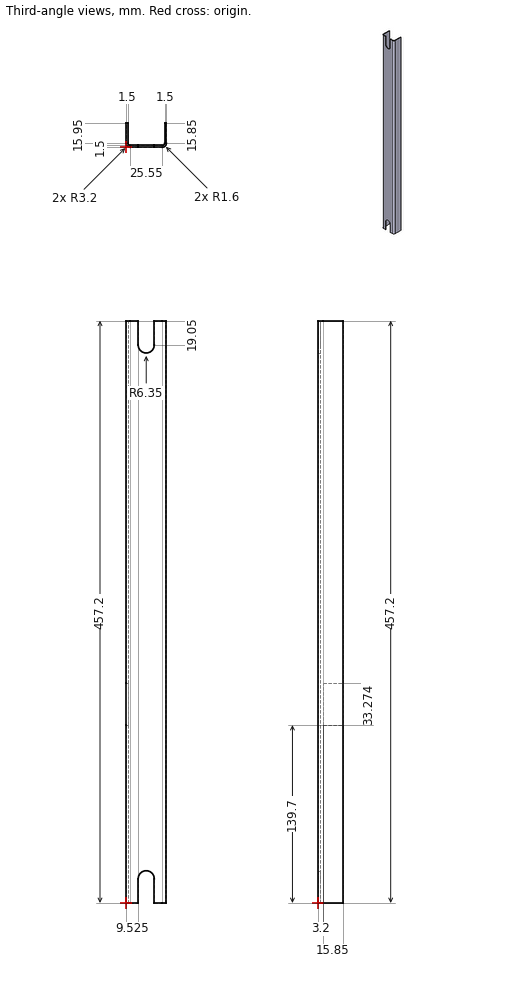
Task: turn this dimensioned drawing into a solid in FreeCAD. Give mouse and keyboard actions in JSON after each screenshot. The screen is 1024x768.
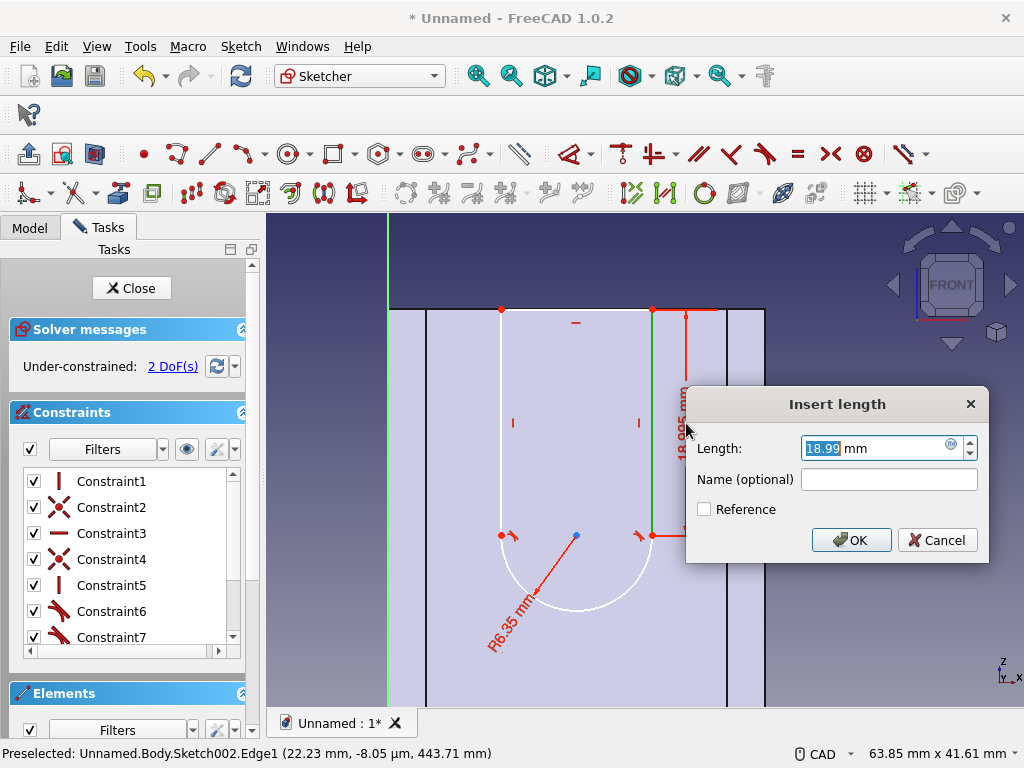
{"action": "type", "text": "19.05"}
{"action": "key", "text": "Return"}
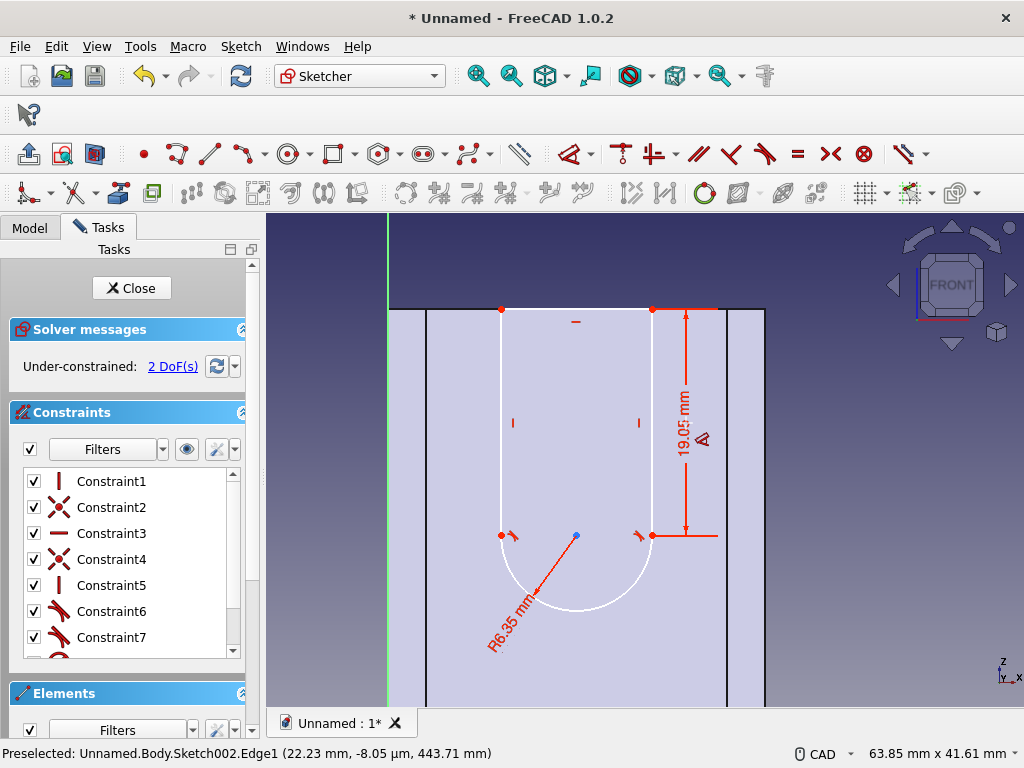
{"action": "left_click", "coordinate": [652, 309]}
{"action": "left_click", "coordinate": [354, 494]}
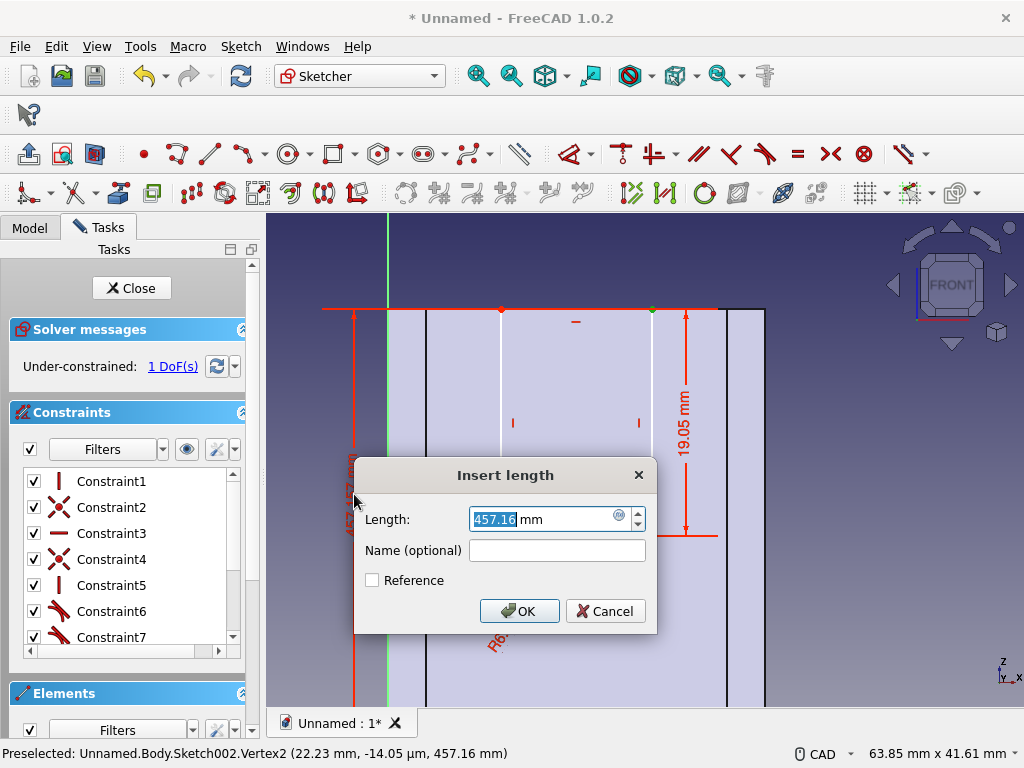
{"action": "type", "text": "457.2"}
{"action": "key", "text": "Return"}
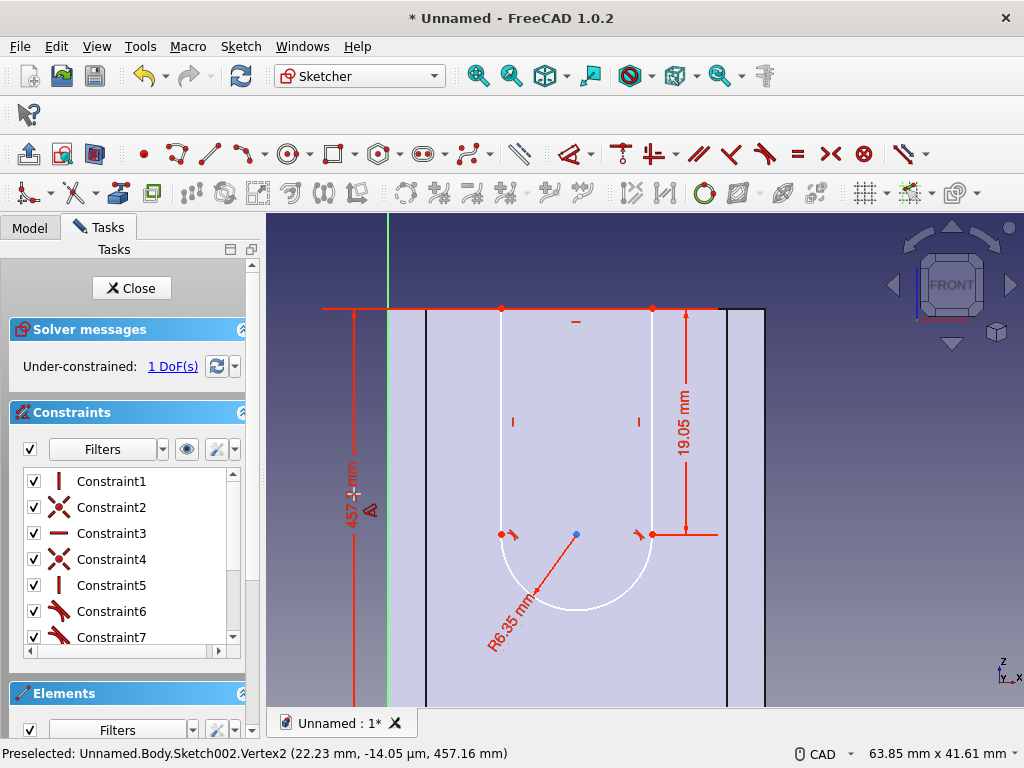
{"action": "left_click", "coordinate": [501, 309]}
{"action": "left_click", "coordinate": [445, 275]}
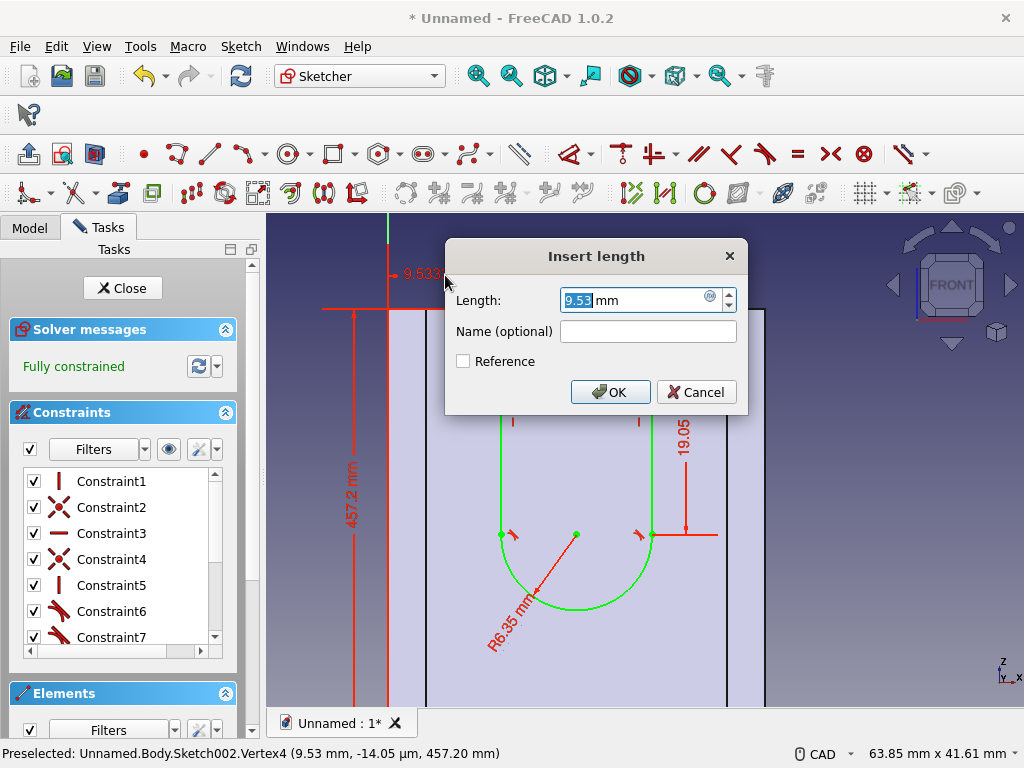
{"action": "type", "text": "9.525"}
{"action": "key", "text": "Return"}
{"action": "key", "text": "Escape"}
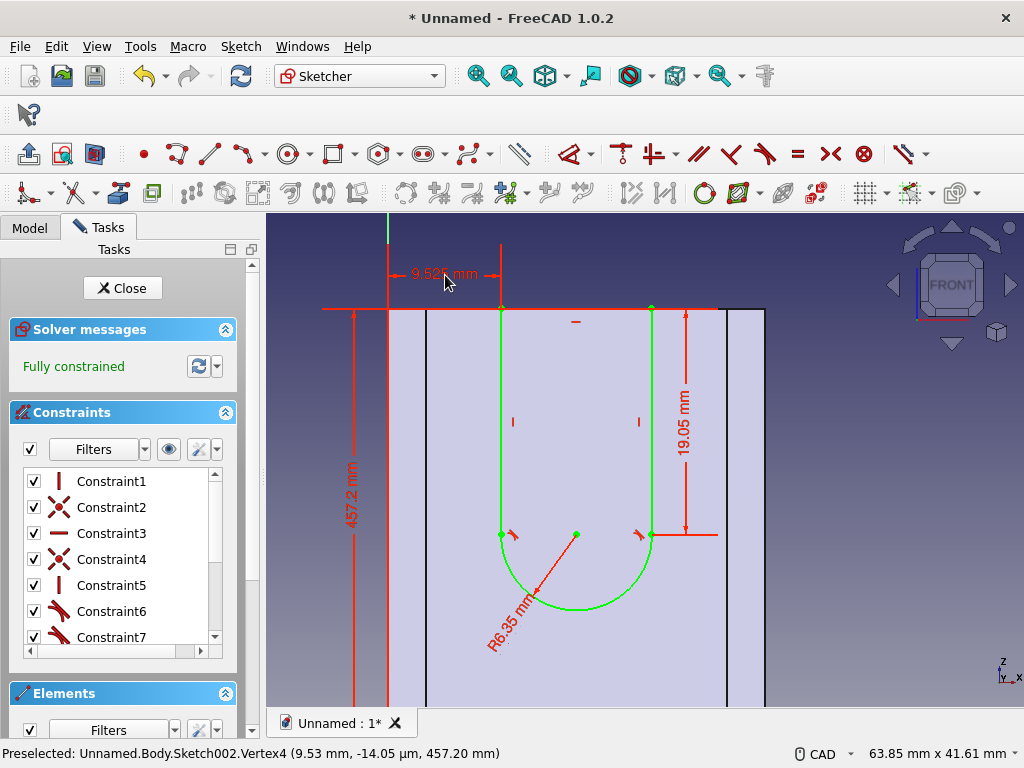
{"action": "left_click", "coordinate": [123, 288]}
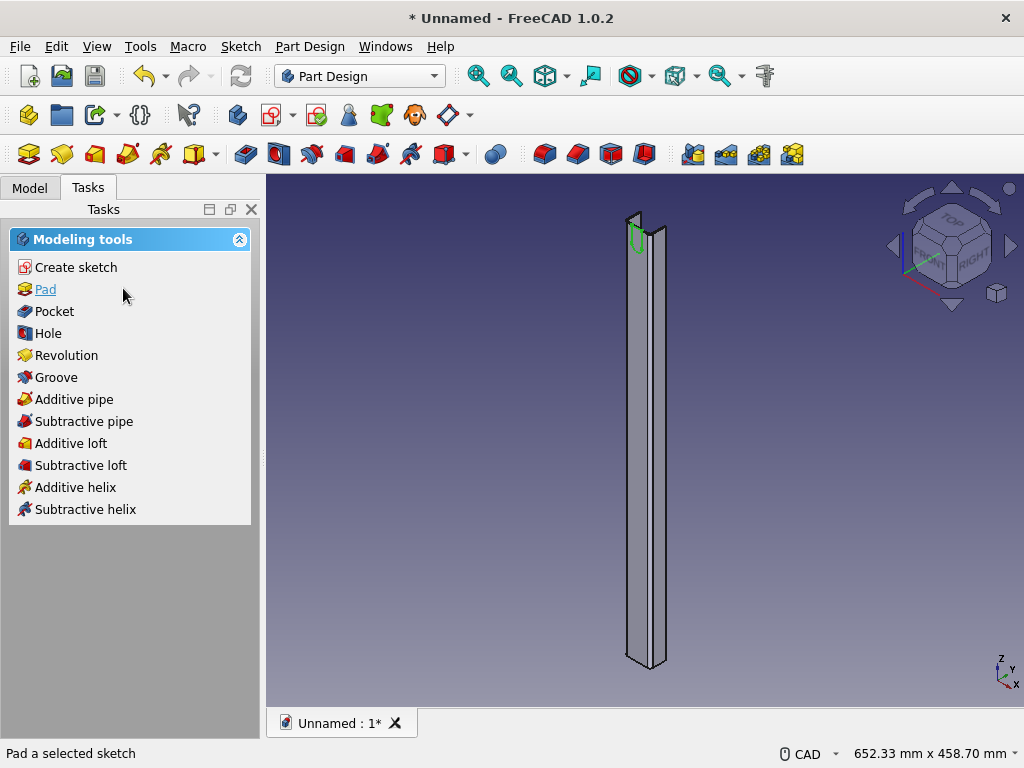
{"action": "left_click", "coordinate": [246, 154]}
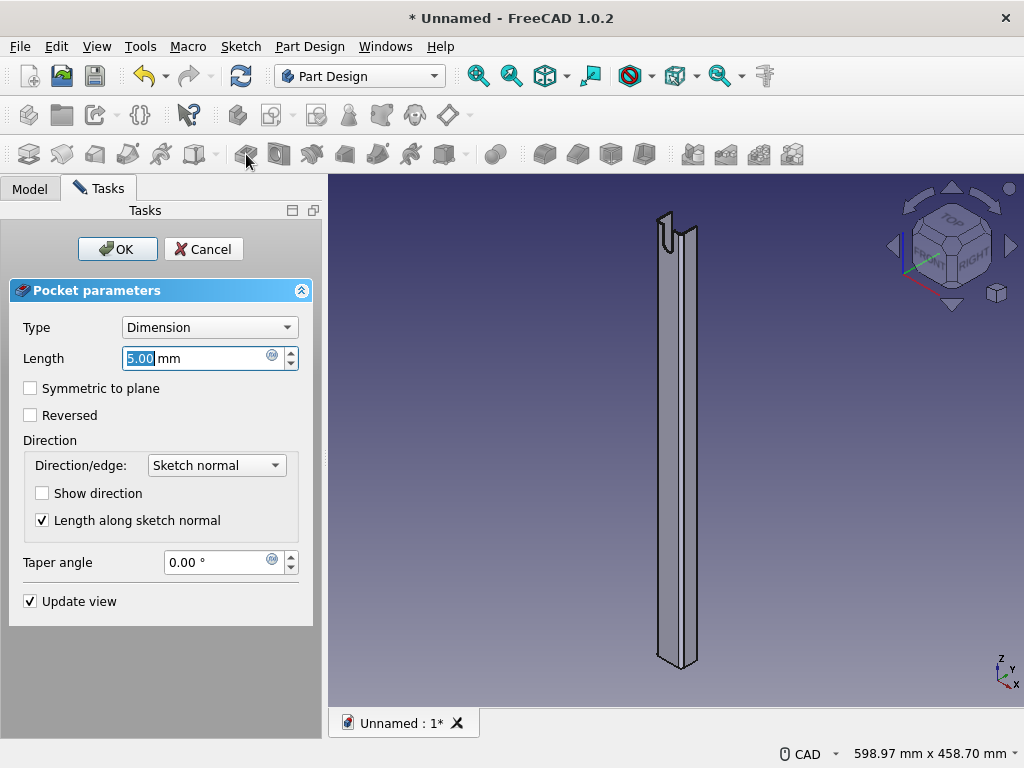
{"action": "left_click", "coordinate": [210, 328]}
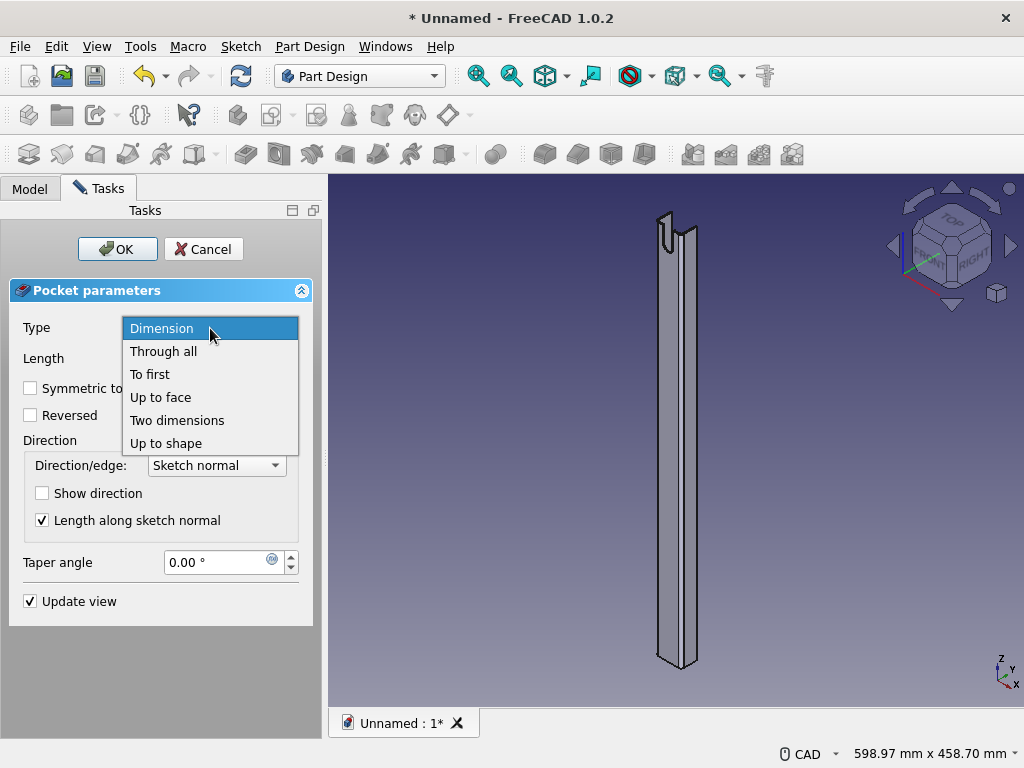
{"action": "left_click", "coordinate": [208, 352]}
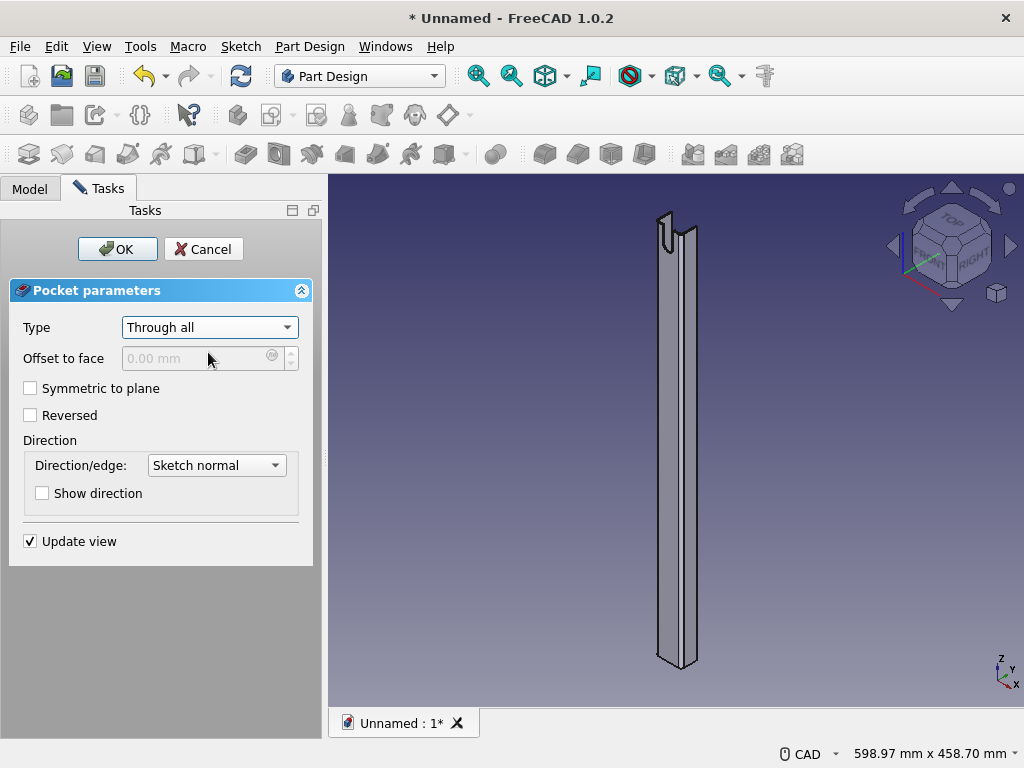
{"action": "left_click", "coordinate": [118, 249]}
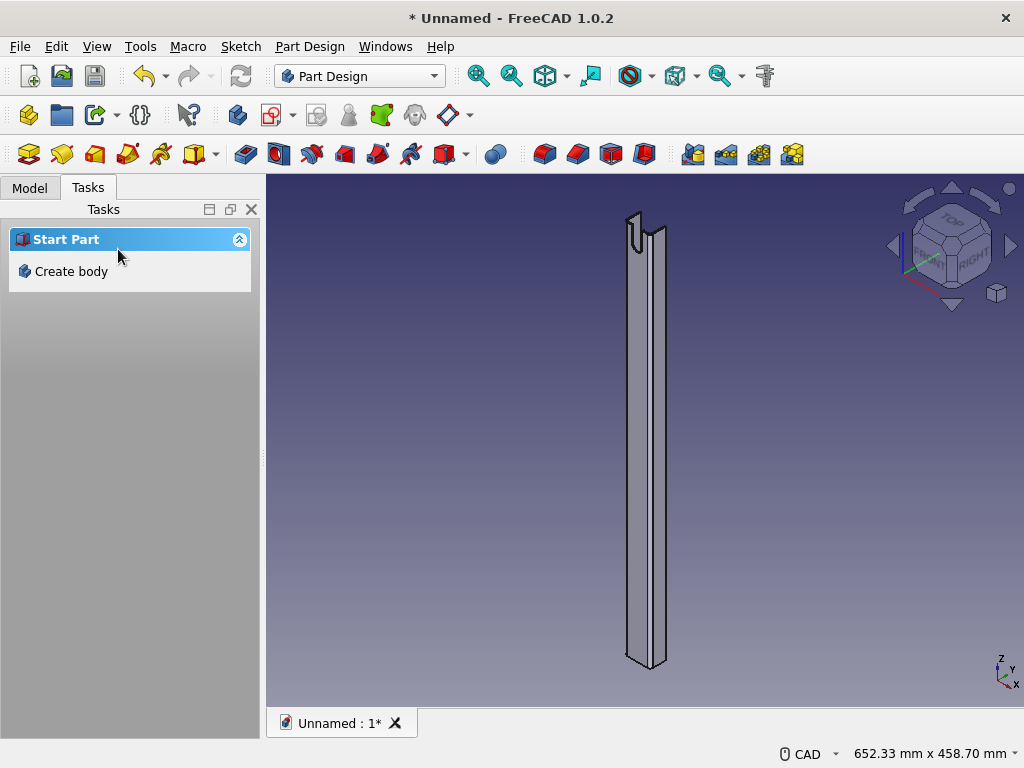
{"action": "left_click", "coordinate": [30, 188]}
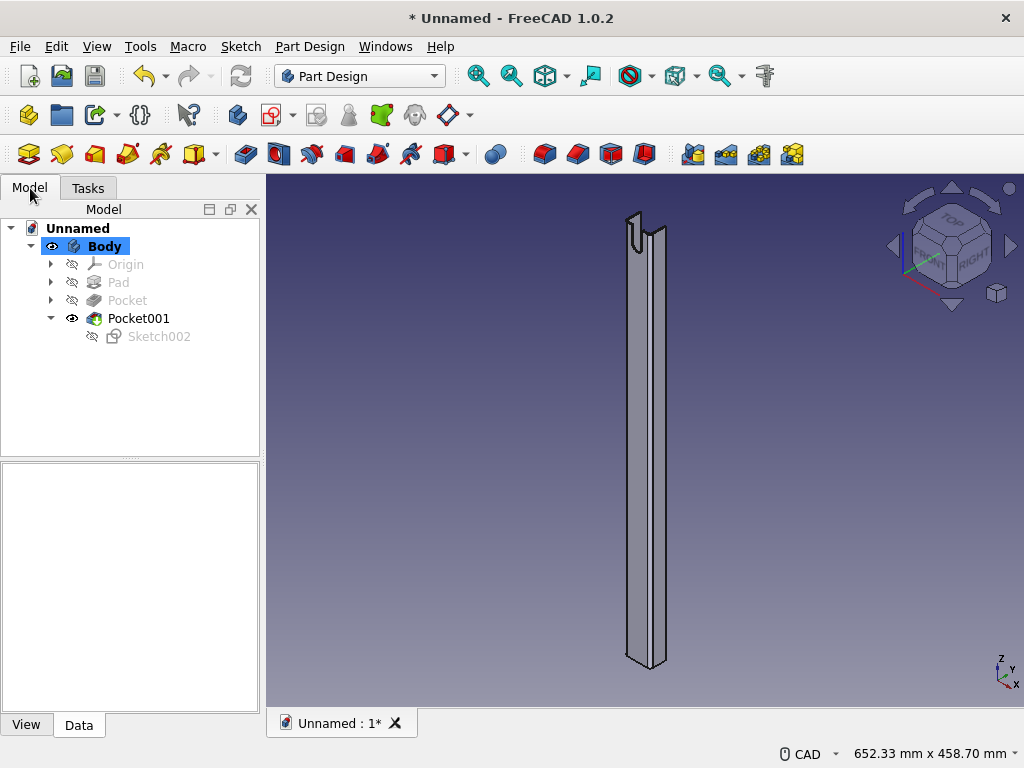
{"action": "left_click", "coordinate": [51, 264]}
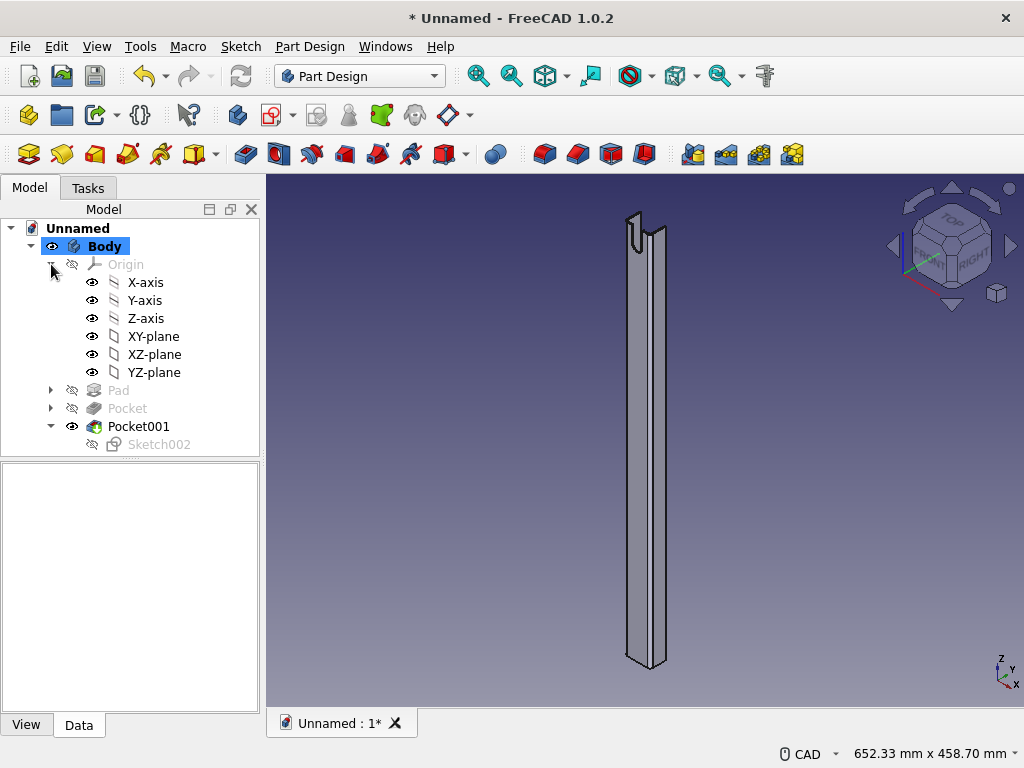
{"action": "left_click", "coordinate": [137, 336]}